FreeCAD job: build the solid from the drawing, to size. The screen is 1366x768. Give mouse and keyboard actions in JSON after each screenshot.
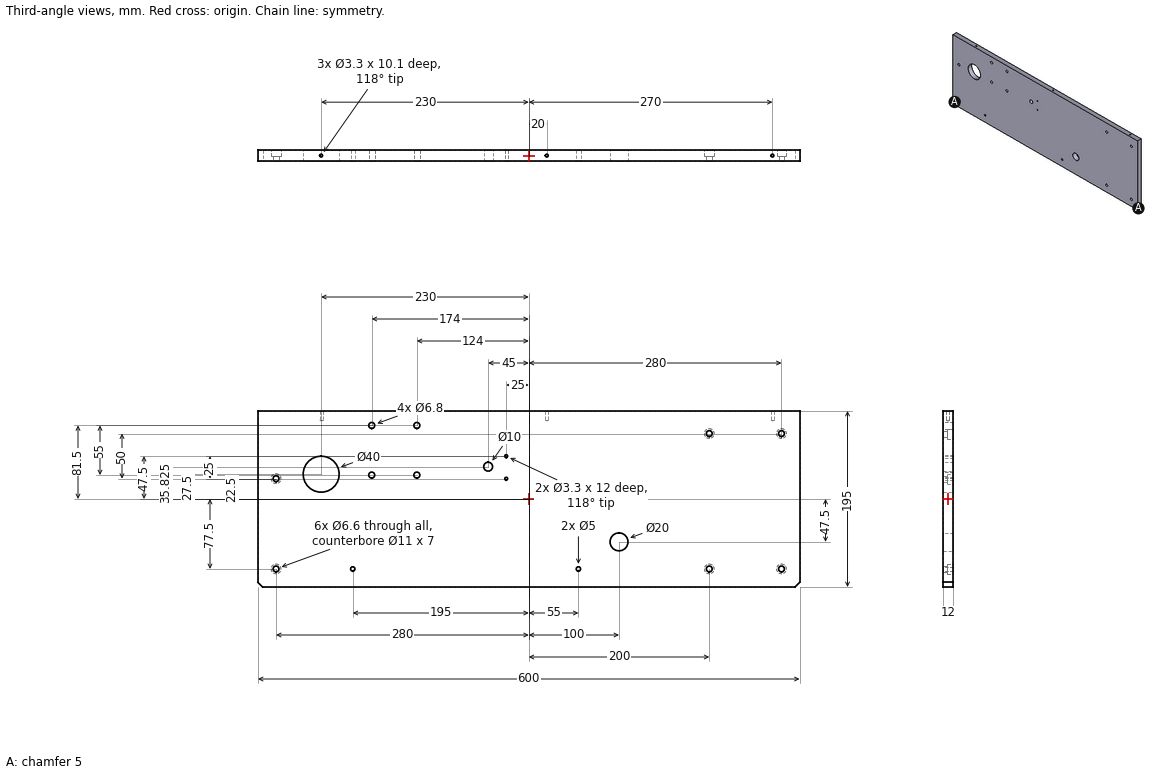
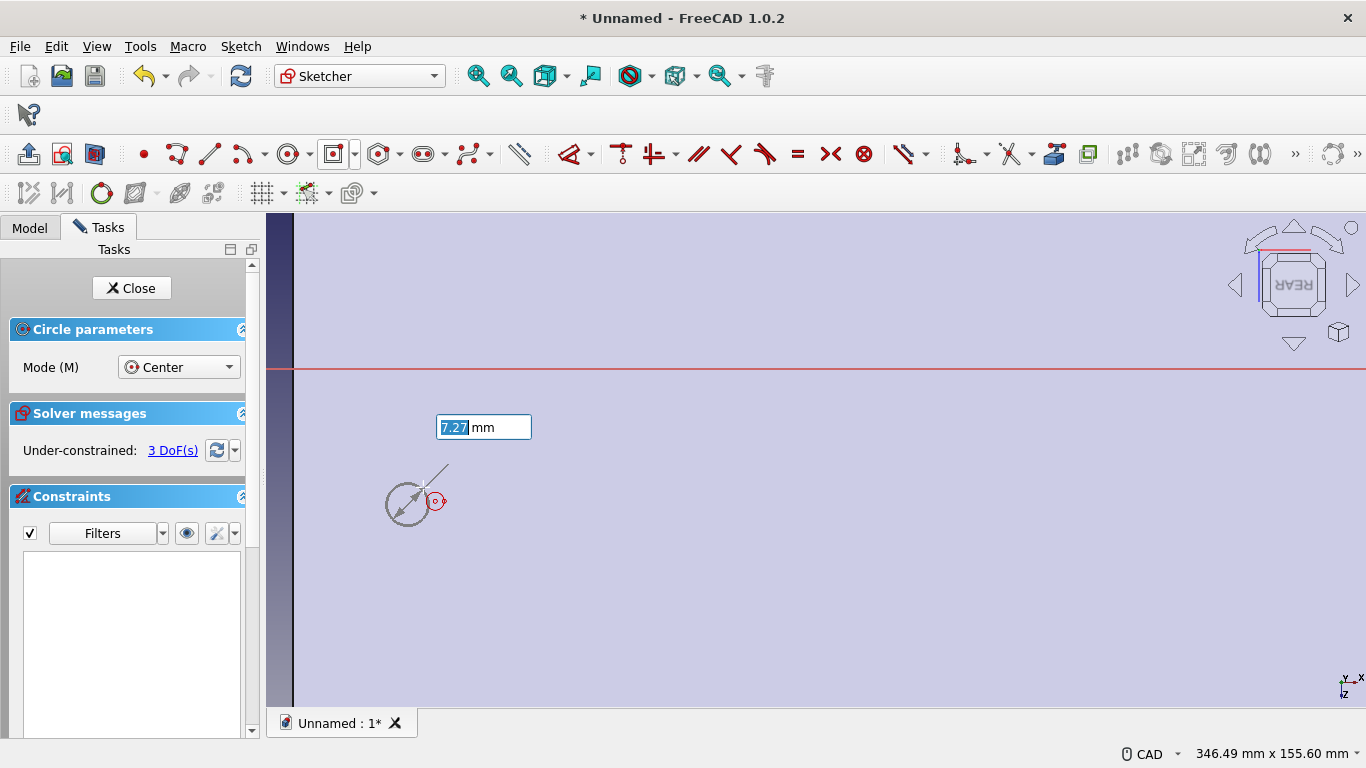
{"action": "left_click", "coordinate": [423, 485]}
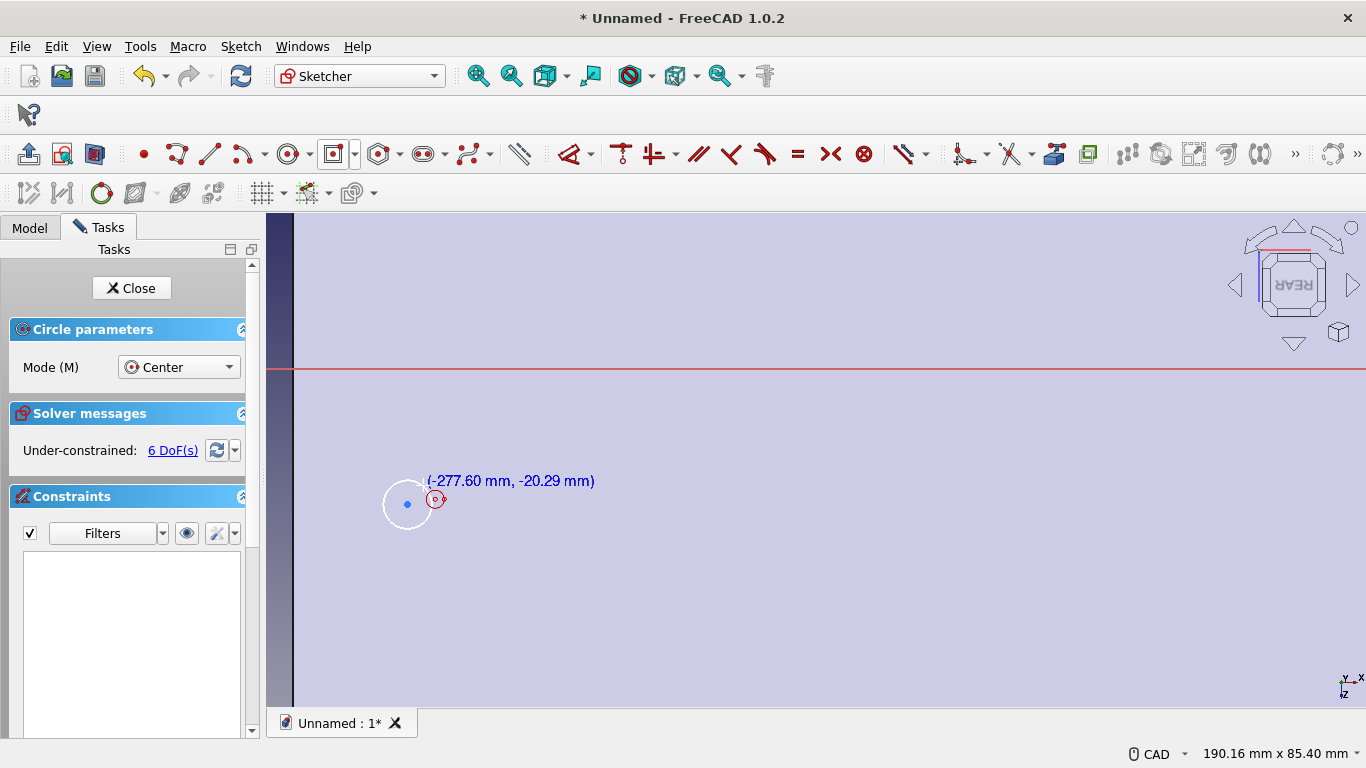
{"action": "scroll", "coordinate": [423, 487], "scroll_direction": "down", "scroll_amount": 8}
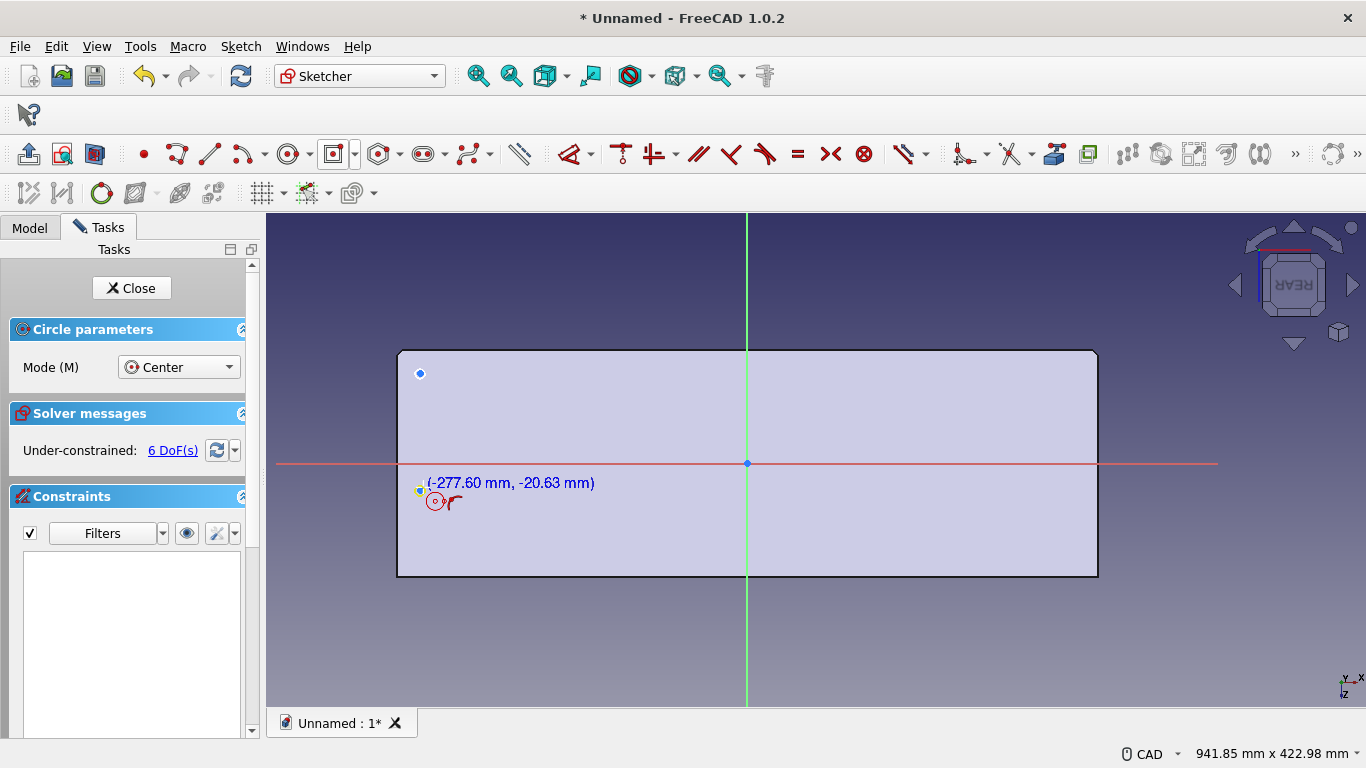
{"action": "scroll", "coordinate": [981, 373], "scroll_direction": "up", "scroll_amount": 9}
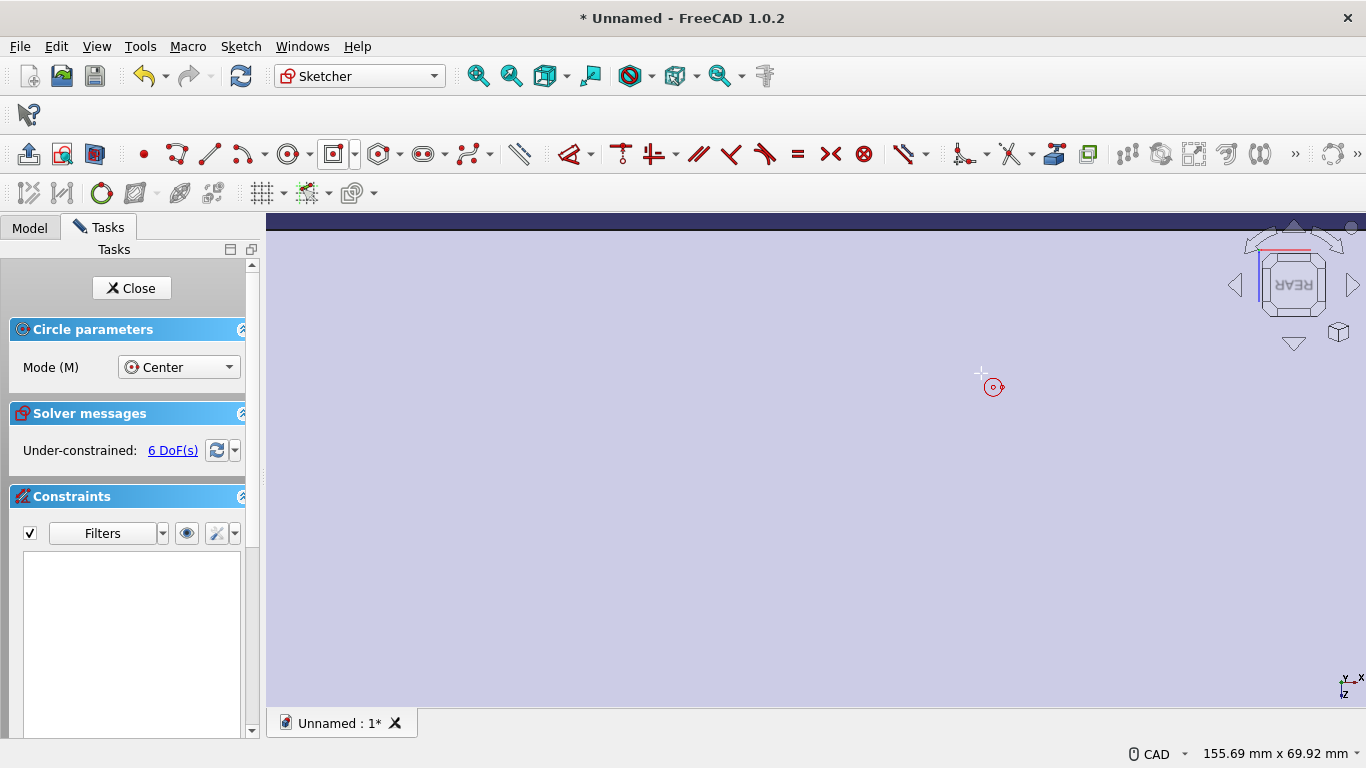
{"action": "scroll", "coordinate": [982, 373], "scroll_direction": "down", "scroll_amount": 9}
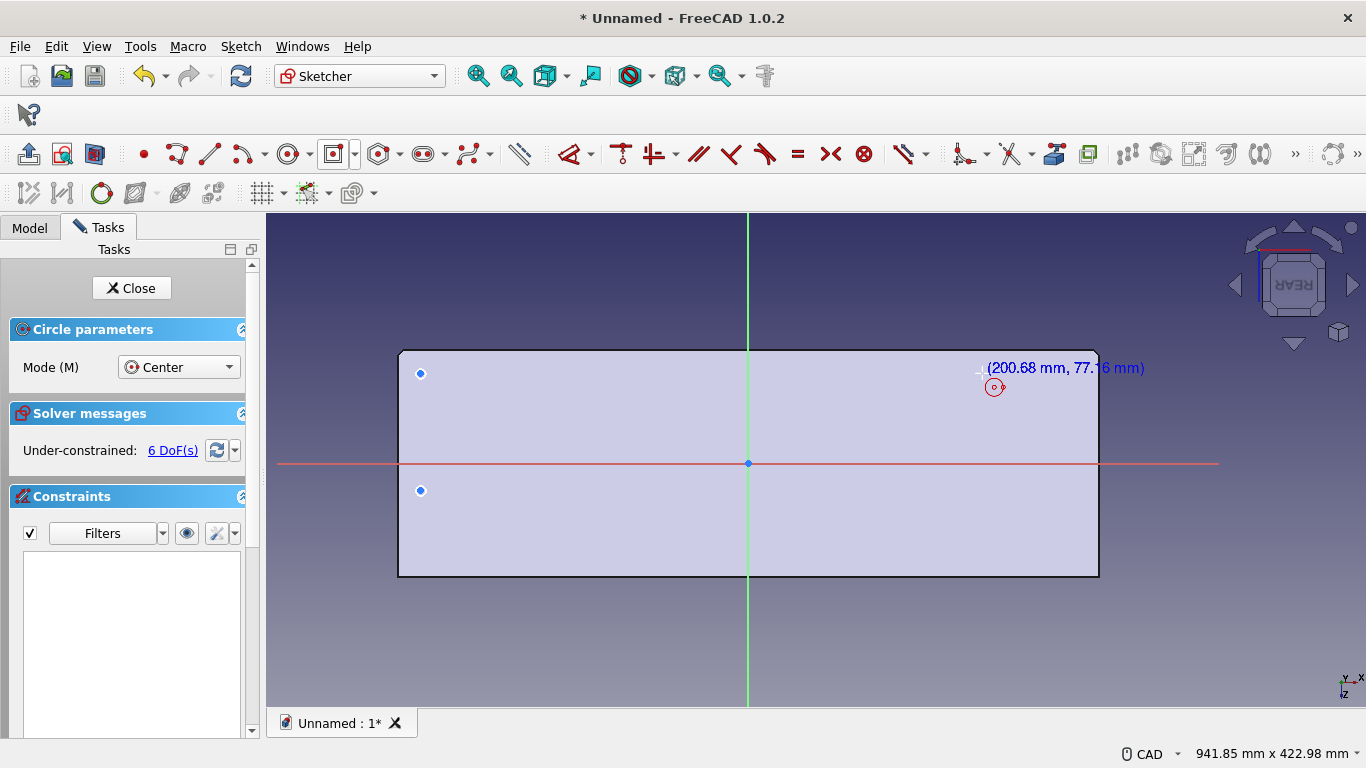
{"action": "left_click", "coordinate": [982, 373]}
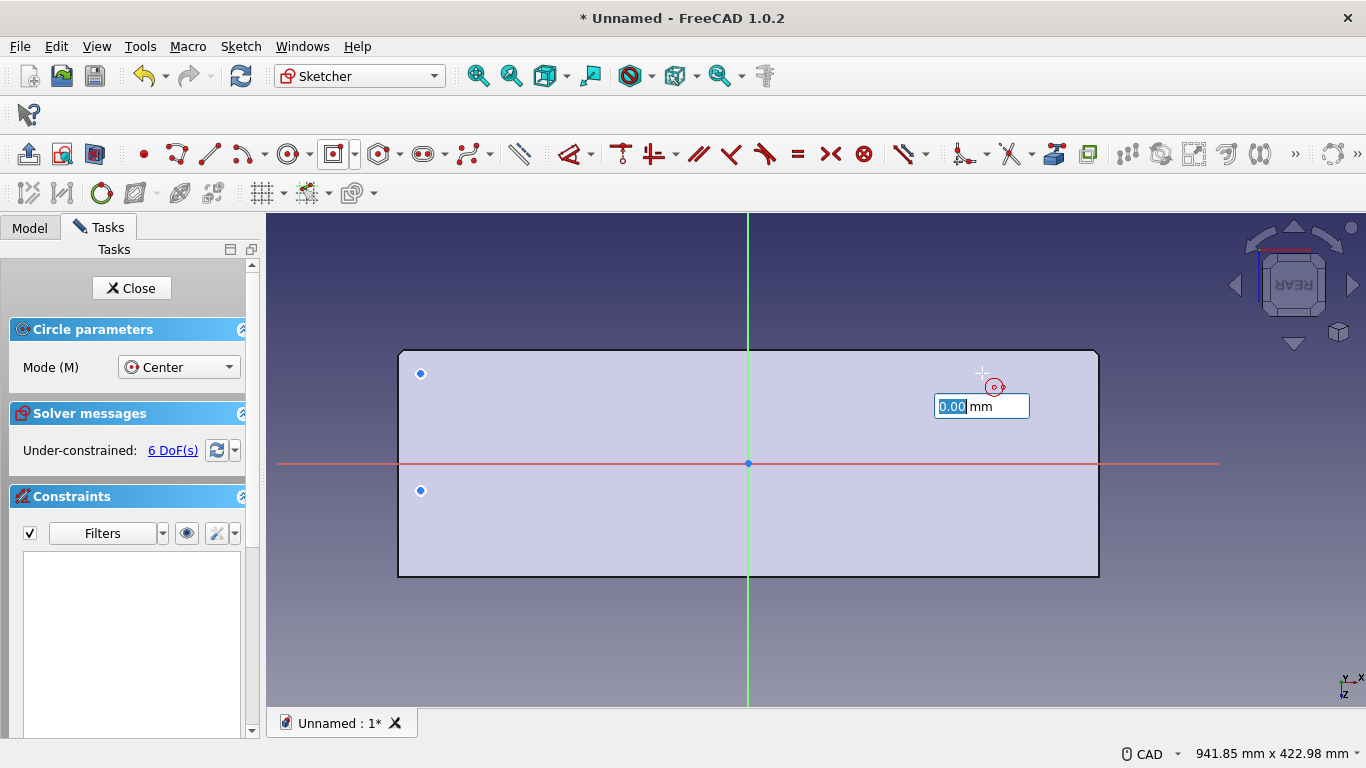
{"action": "scroll", "coordinate": [984, 370], "scroll_direction": "up", "scroll_amount": 8}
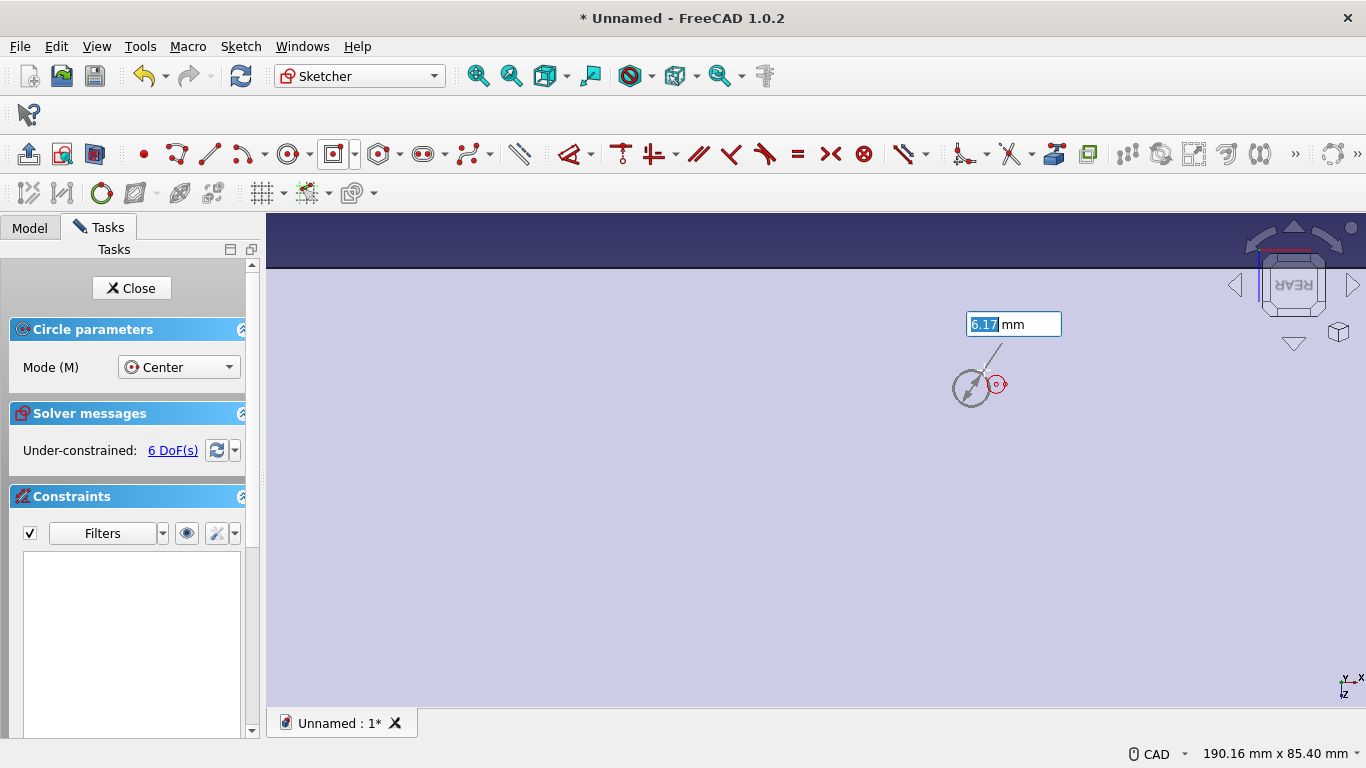
{"action": "left_click", "coordinate": [984, 370]}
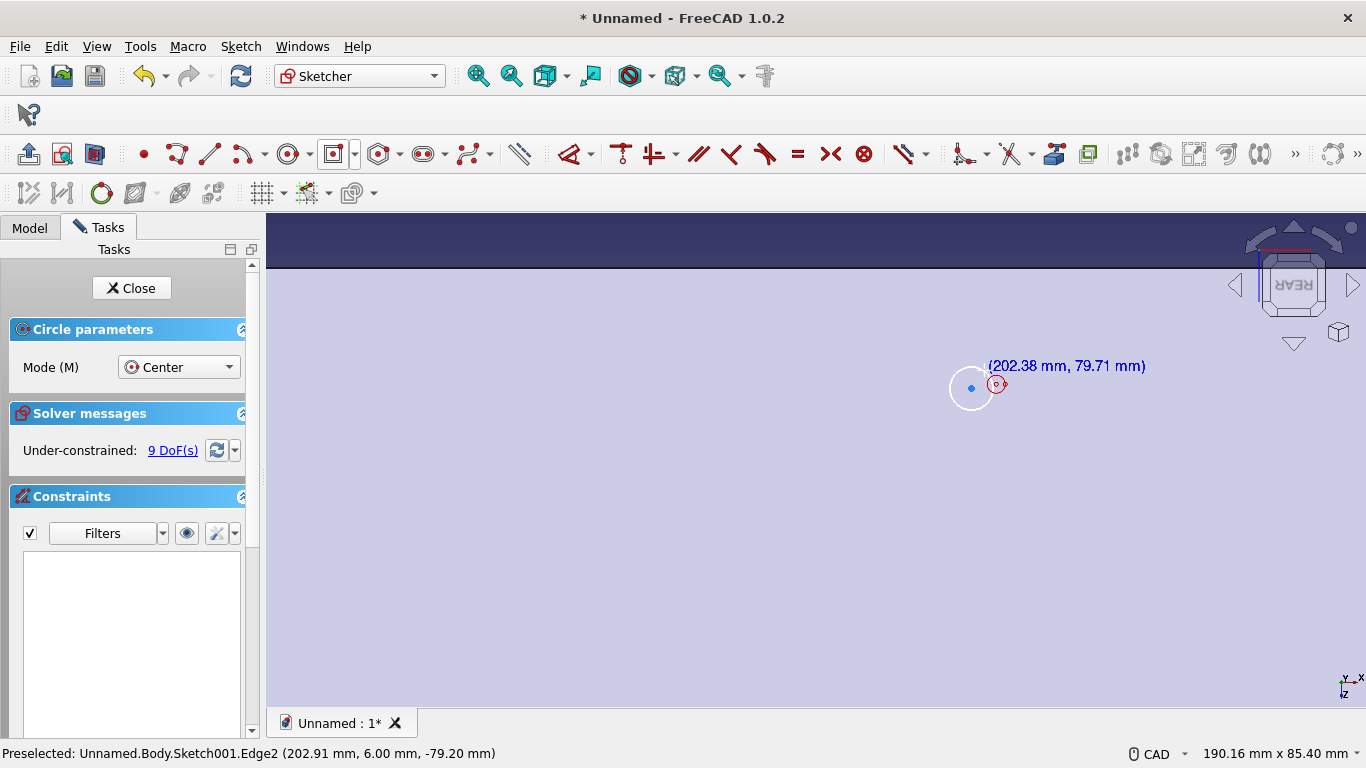
{"action": "scroll", "coordinate": [984, 370], "scroll_direction": "down", "scroll_amount": 8}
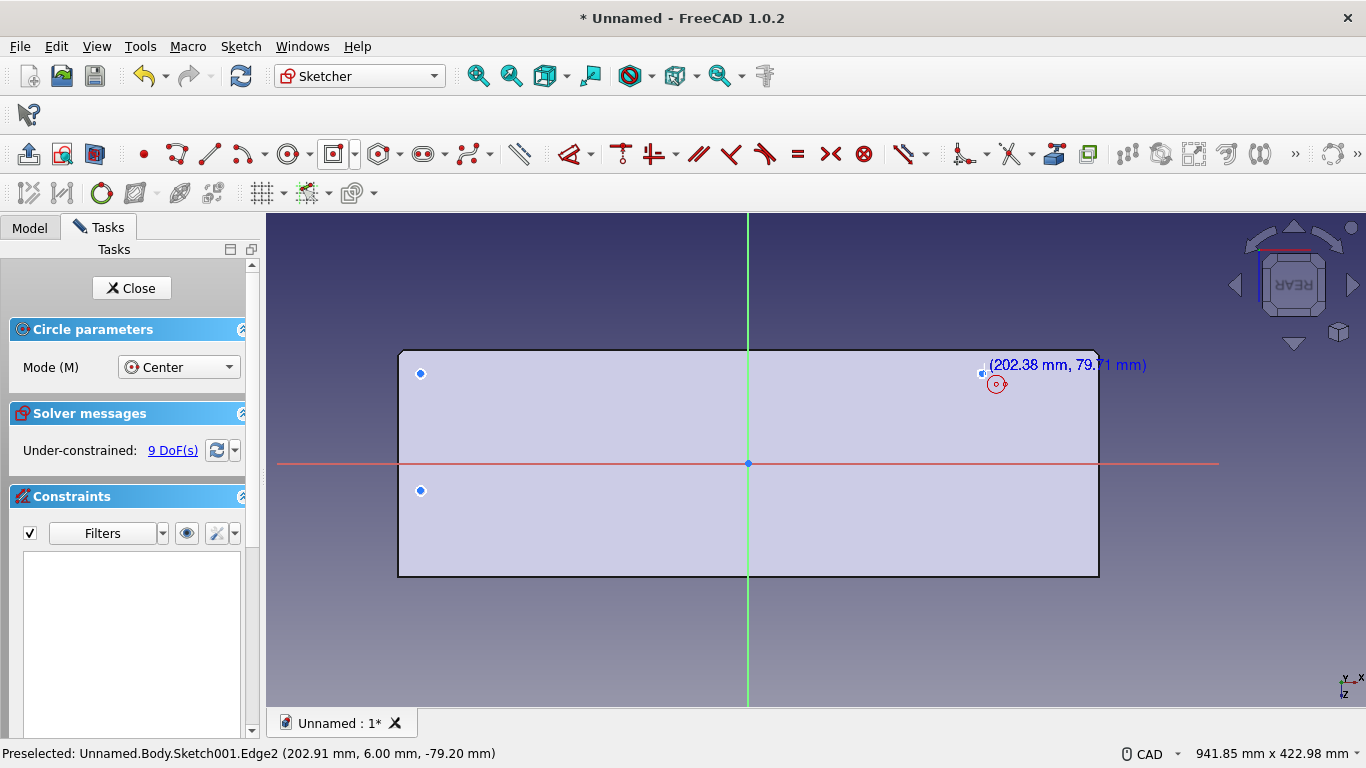
{"action": "scroll", "coordinate": [1075, 373], "scroll_direction": "up", "scroll_amount": 9}